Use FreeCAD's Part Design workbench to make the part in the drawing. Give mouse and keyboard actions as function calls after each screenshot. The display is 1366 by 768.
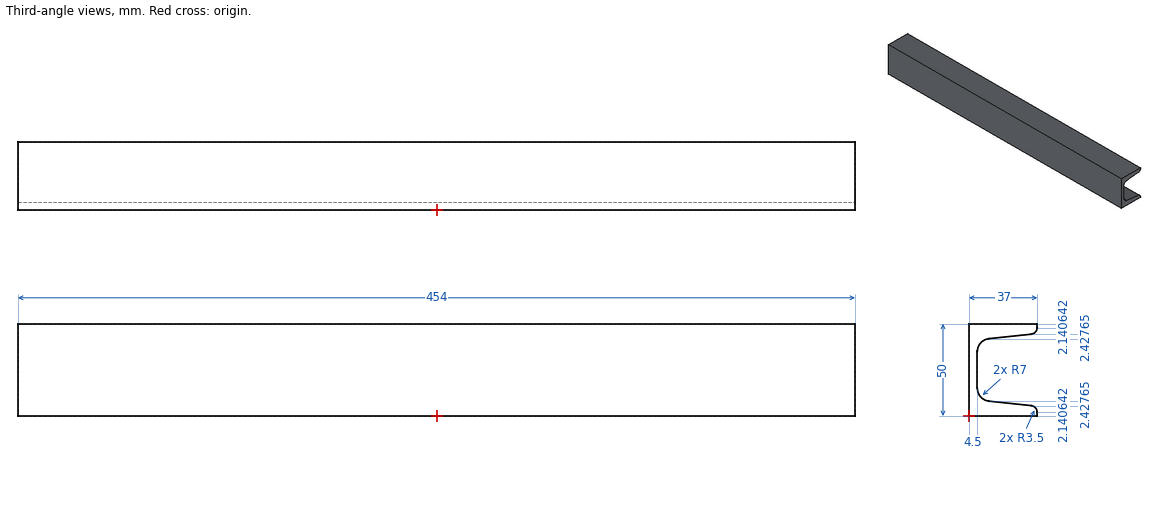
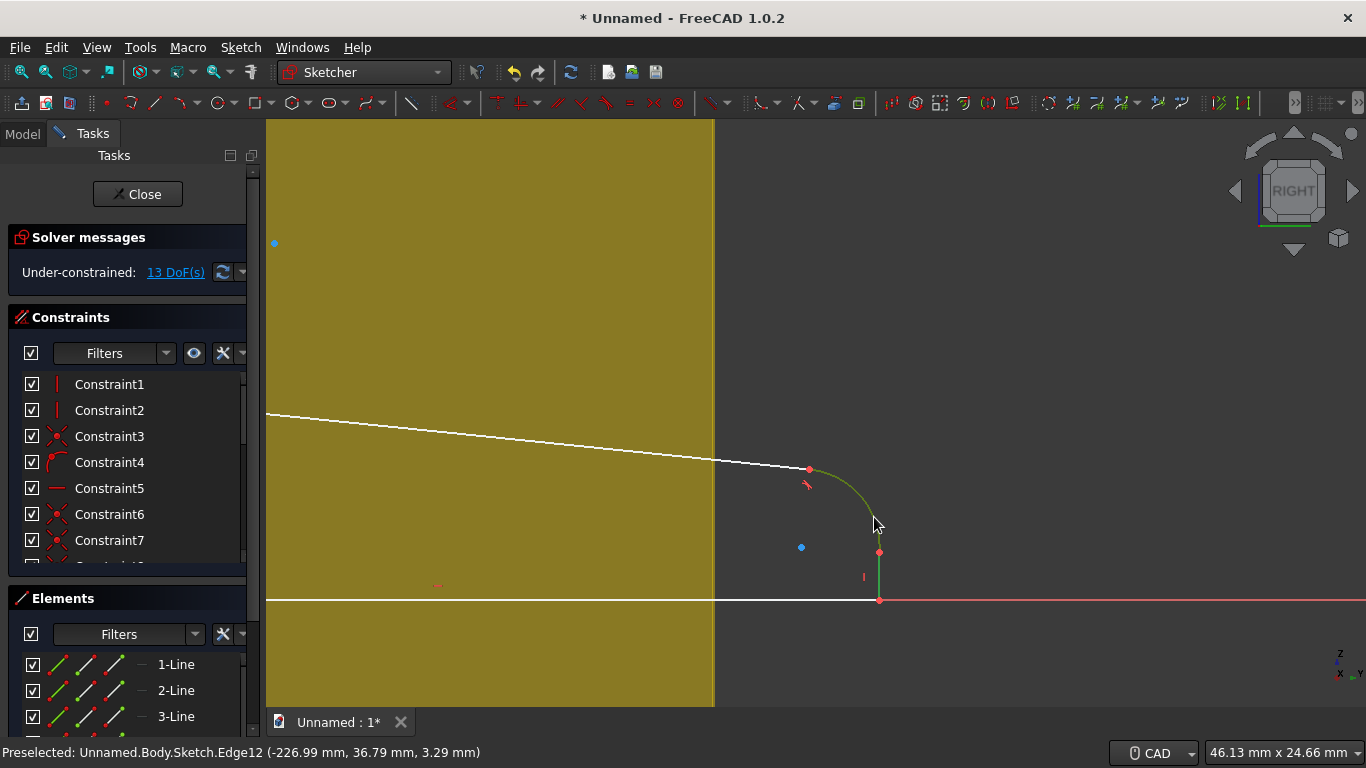
click(606, 104)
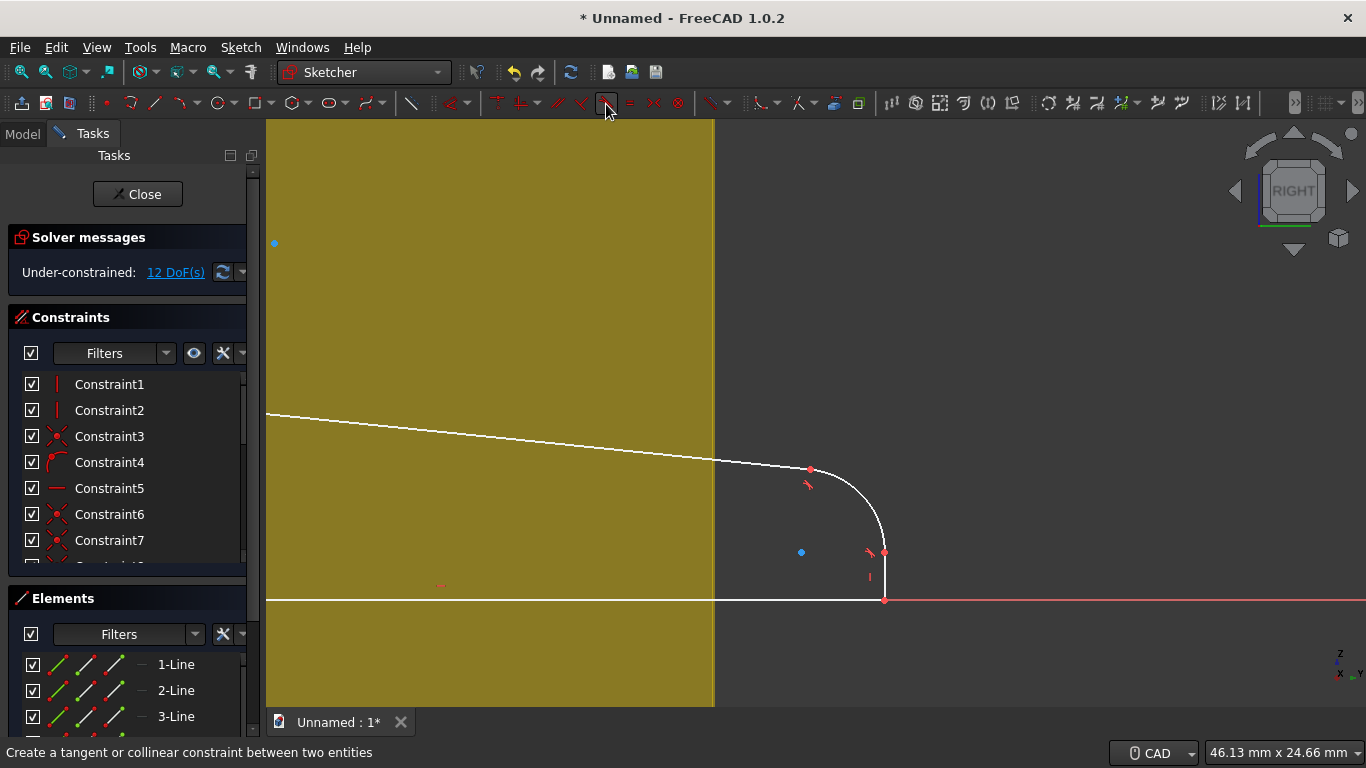
scroll(880, 589, down, 6)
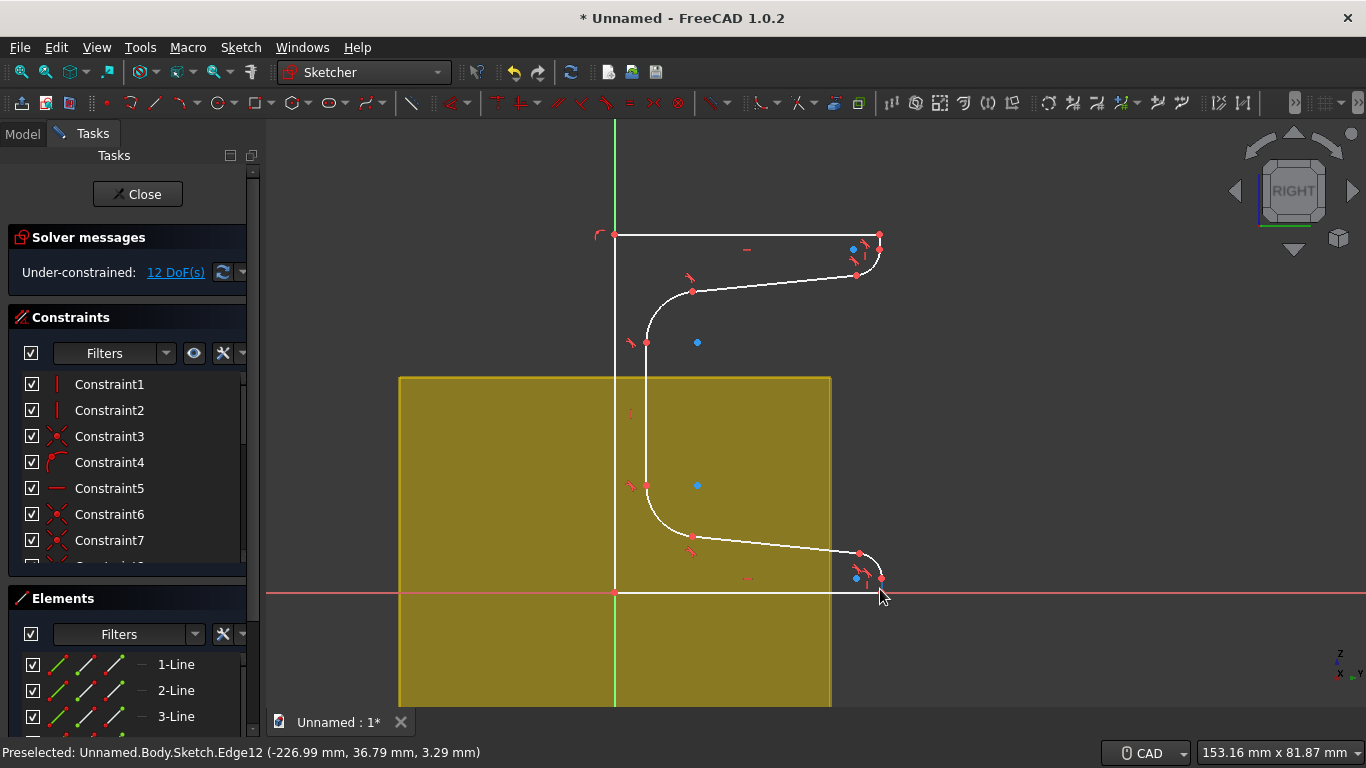
click(651, 507)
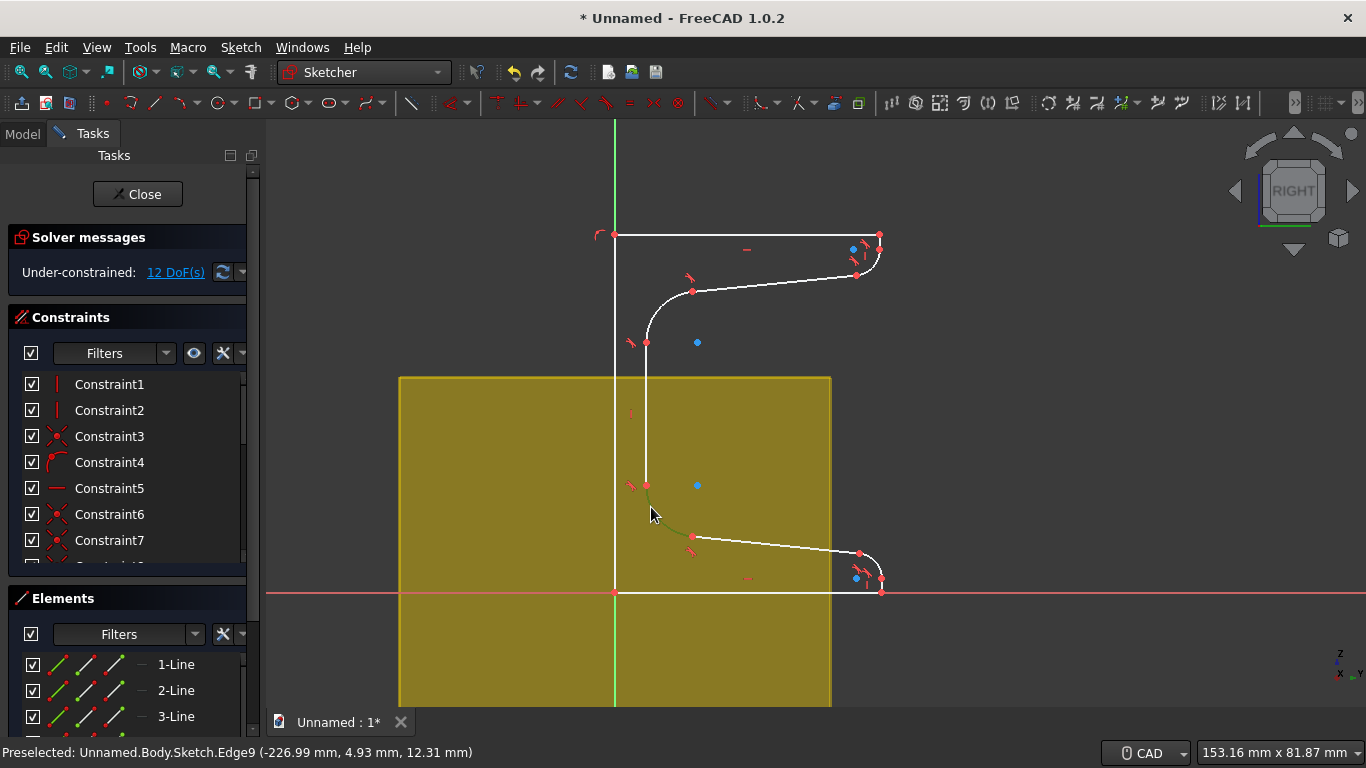
click(671, 299)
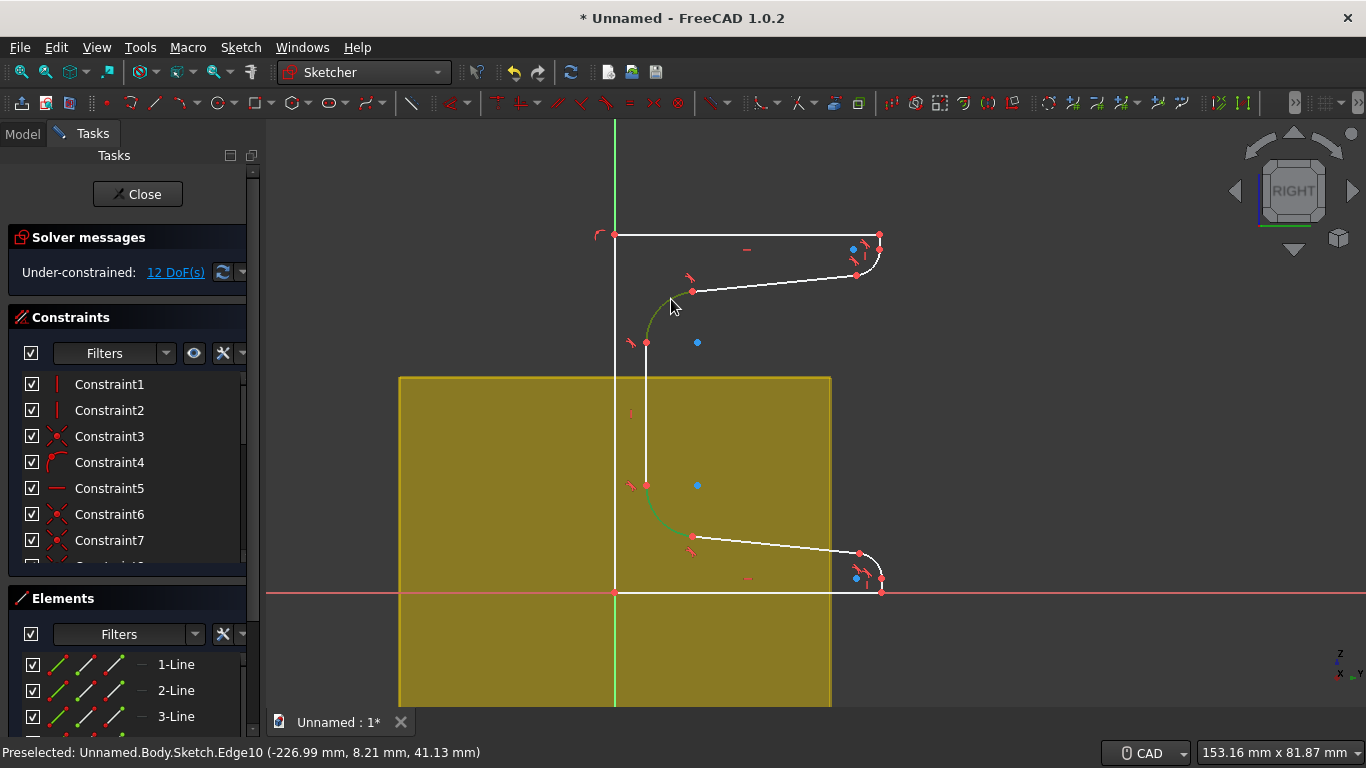
click(630, 104)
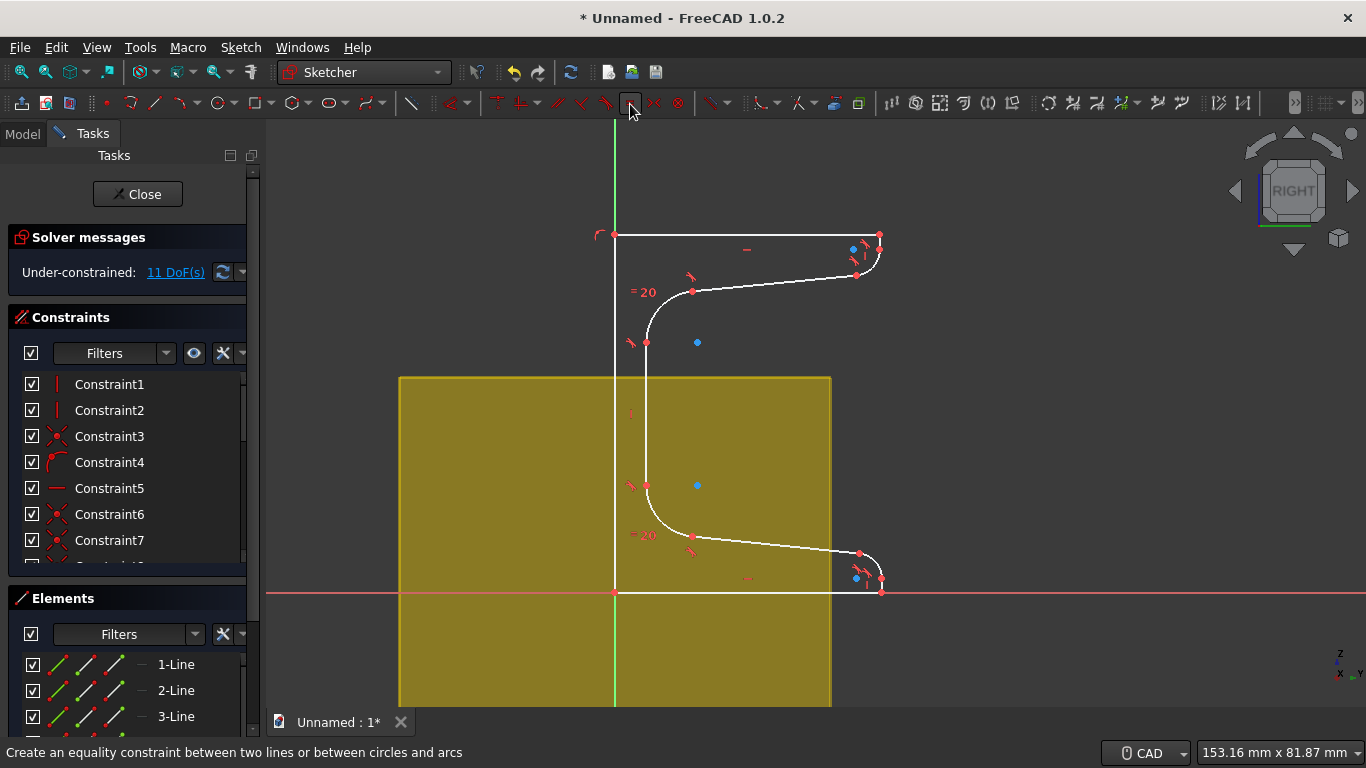
click(867, 272)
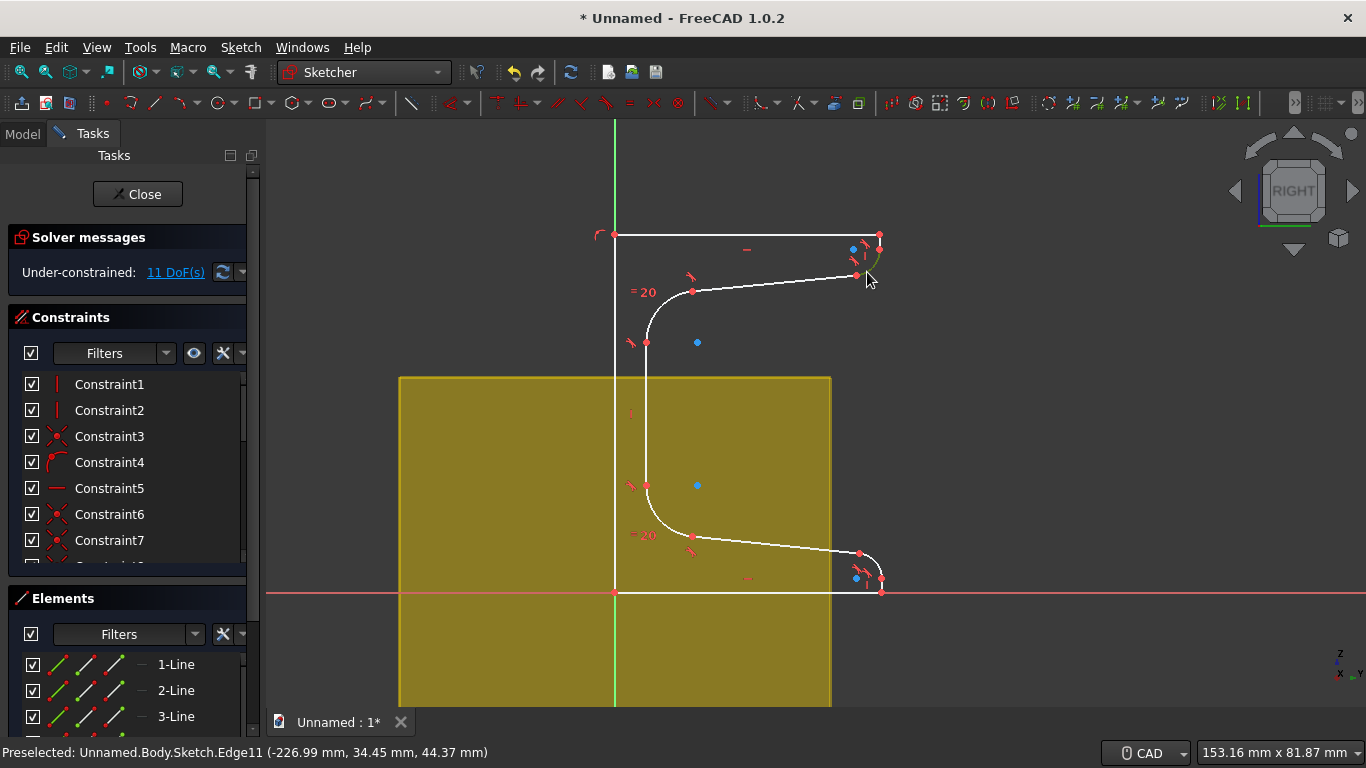
scroll(879, 568, up, 2)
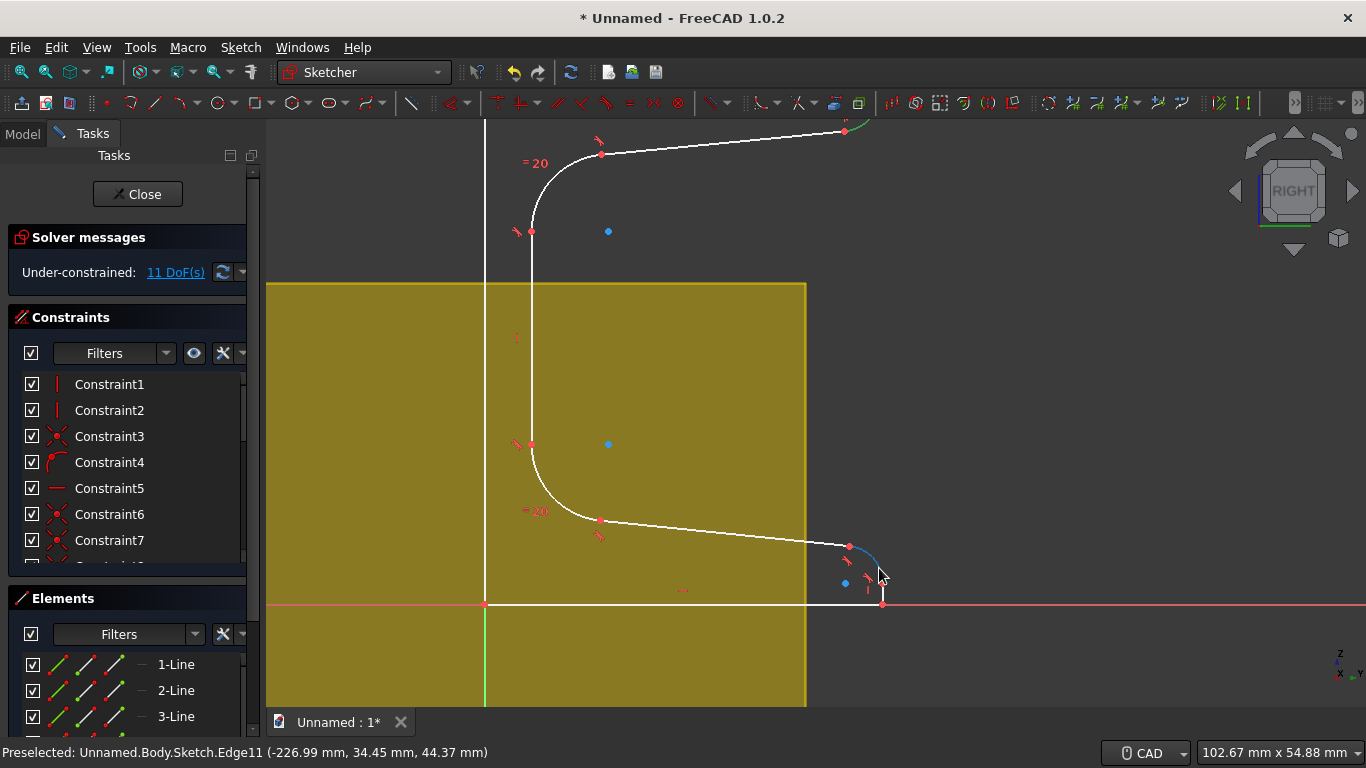
click(879, 567)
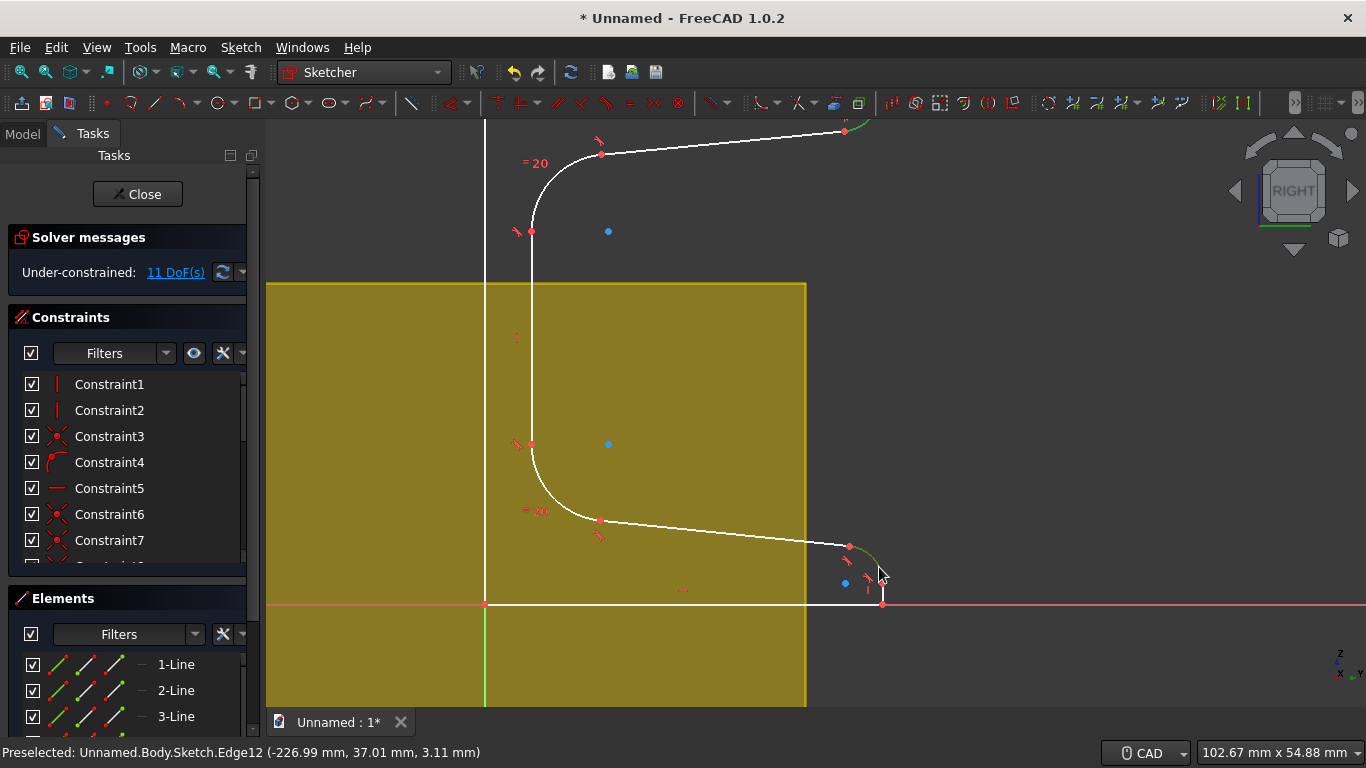
click(630, 104)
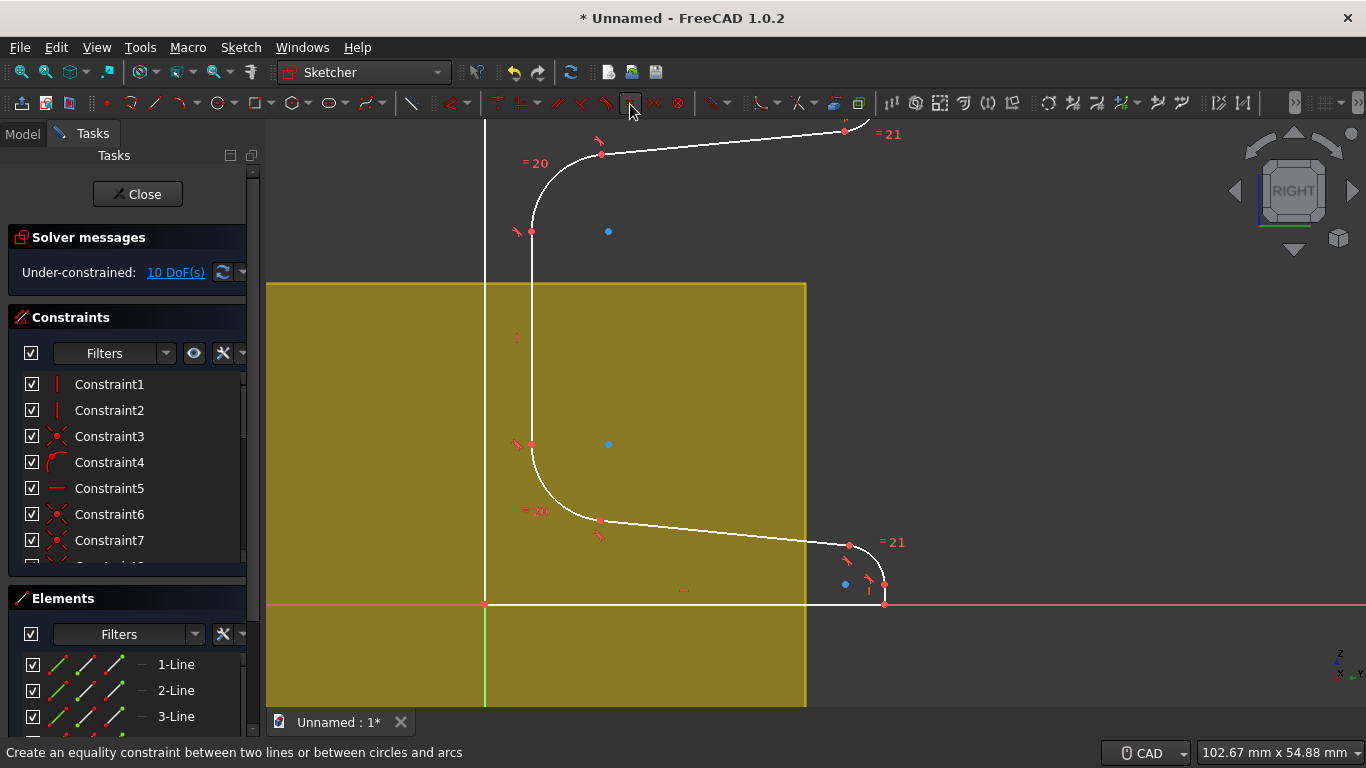
key(d)